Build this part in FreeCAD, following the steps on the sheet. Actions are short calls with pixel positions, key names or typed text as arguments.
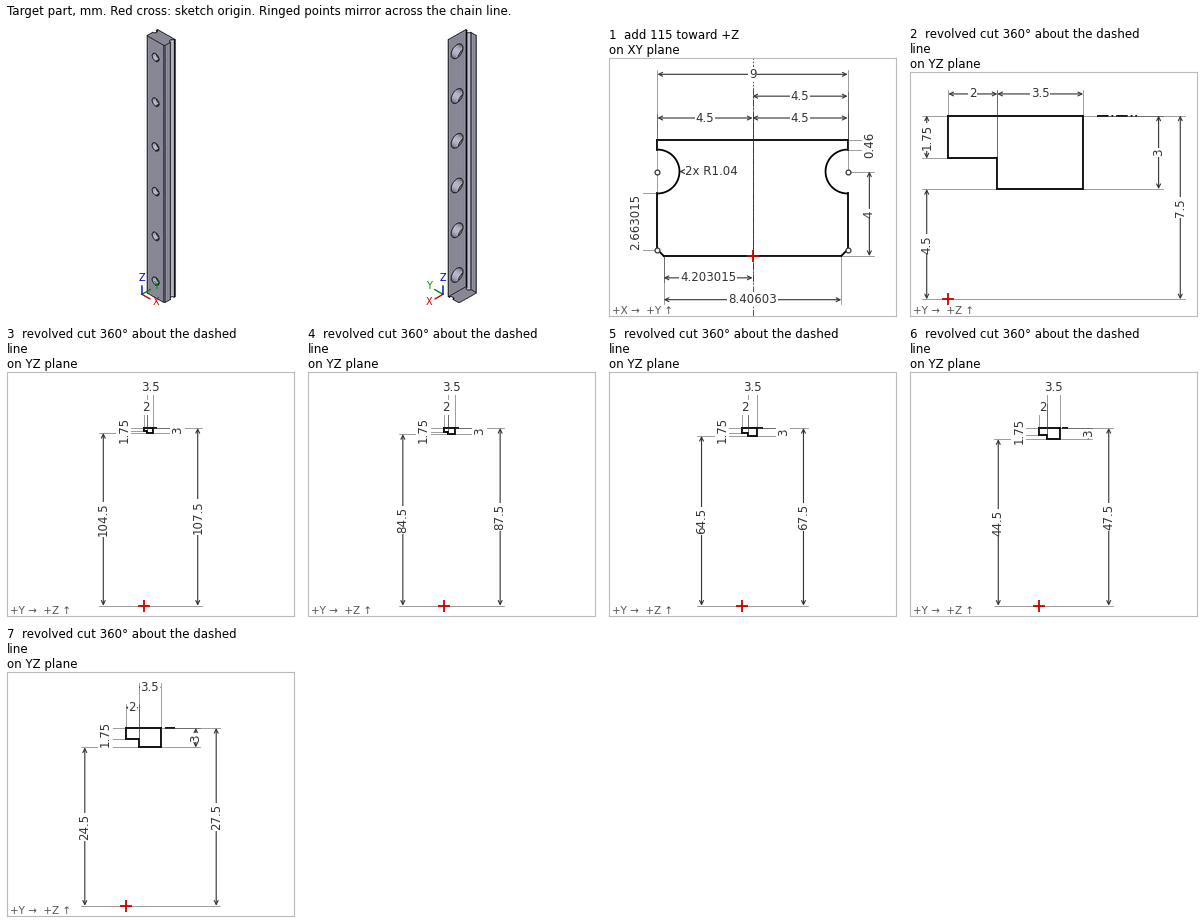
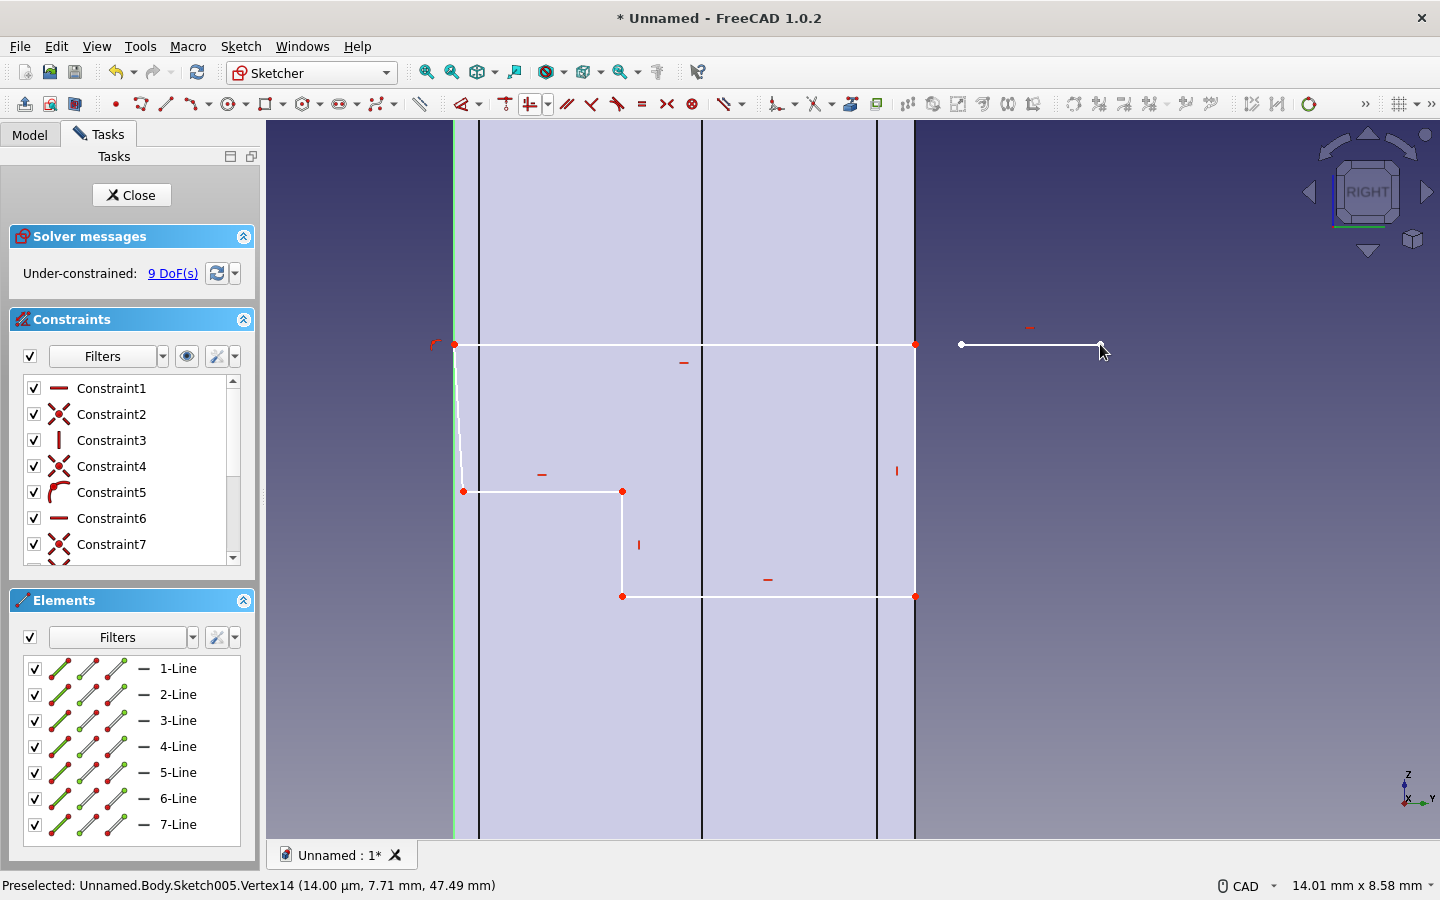
click(1003, 345)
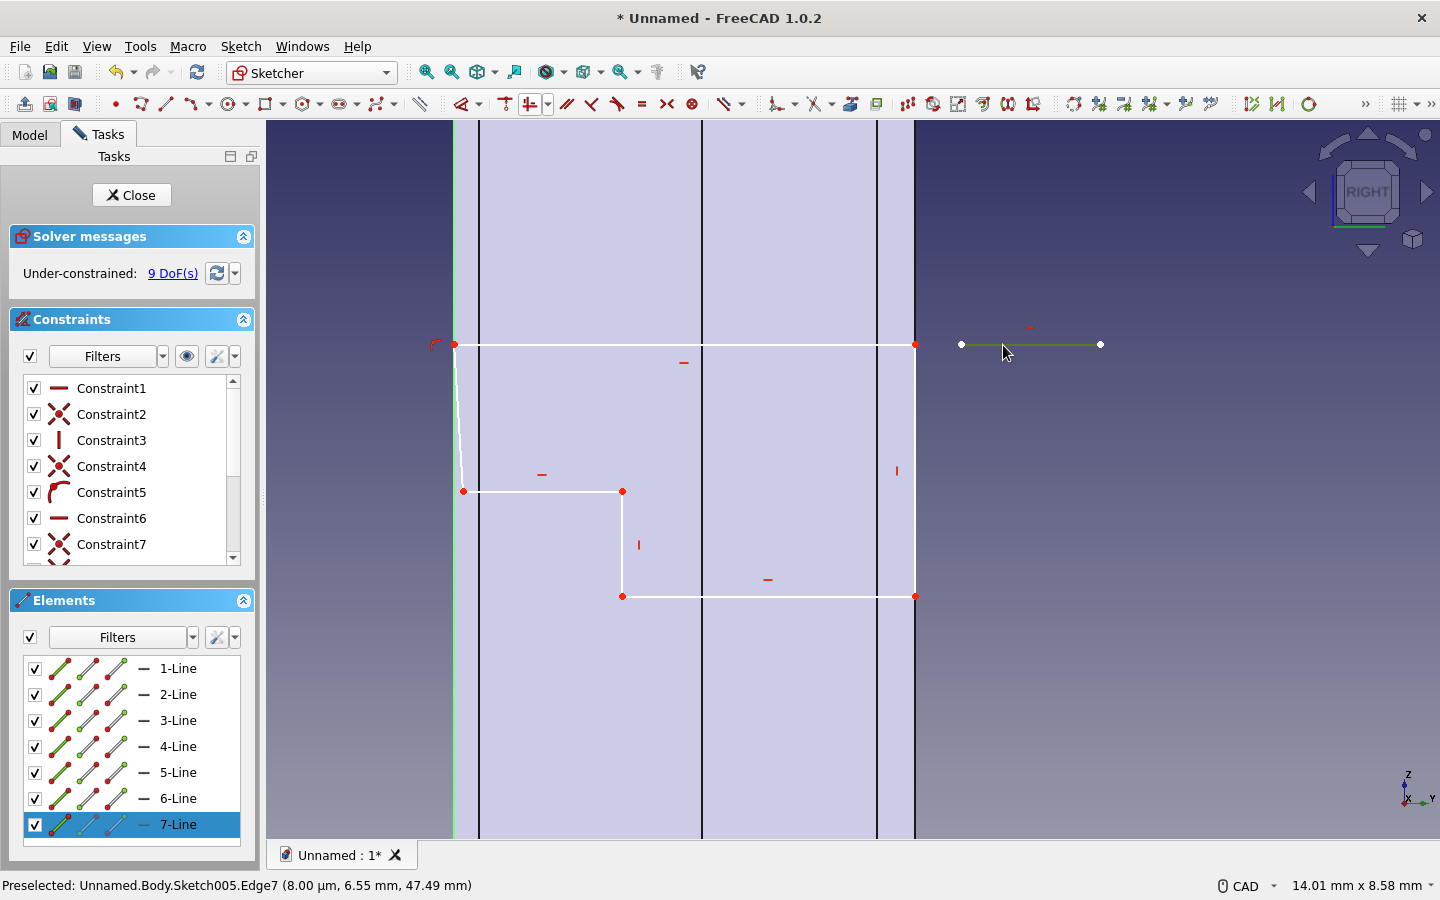
key(g)
key(n)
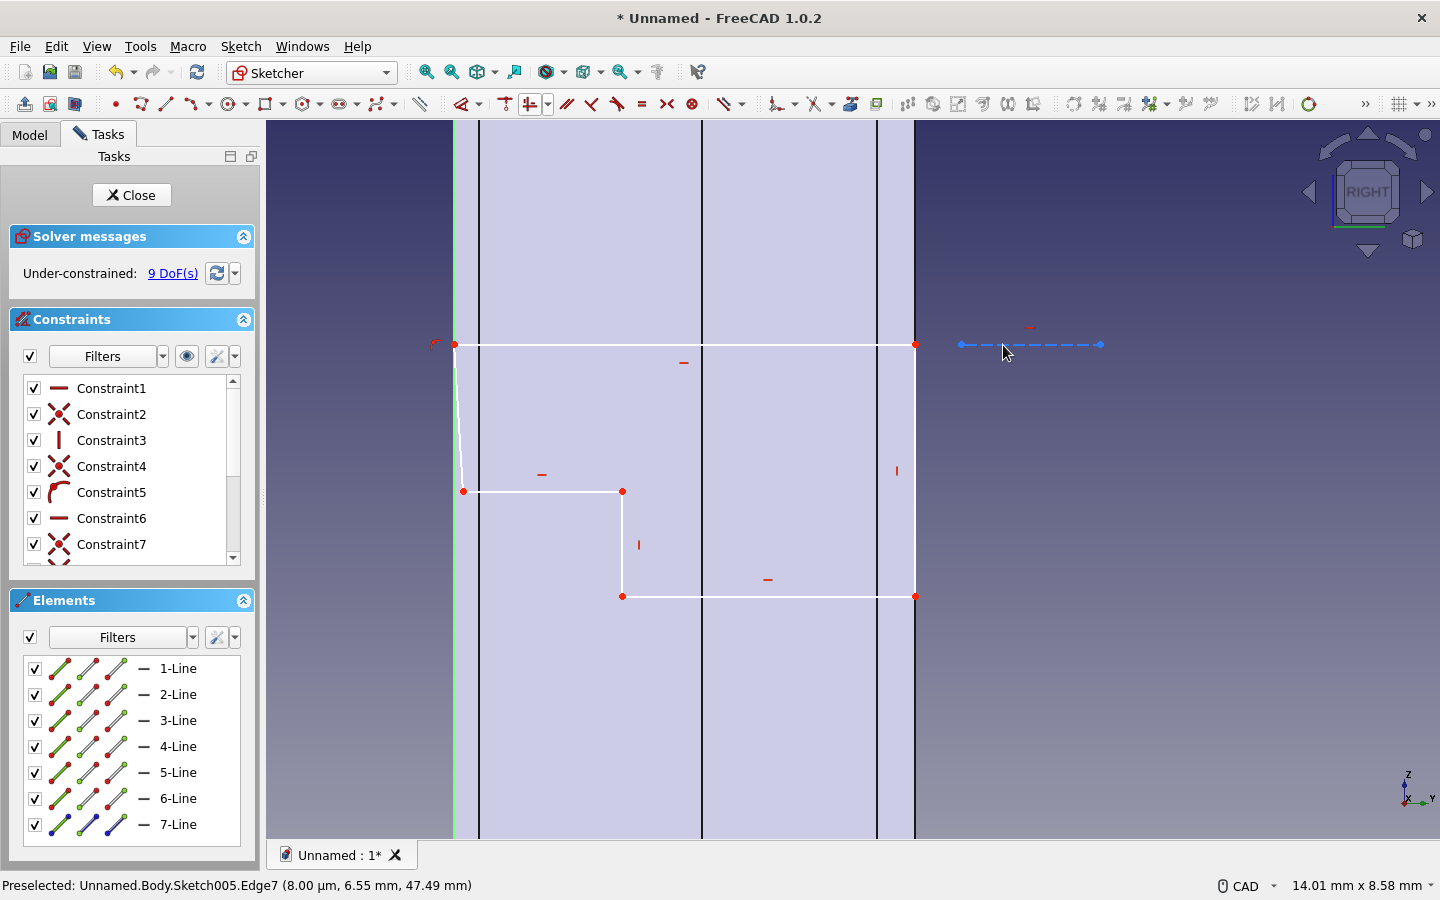
click(457, 389)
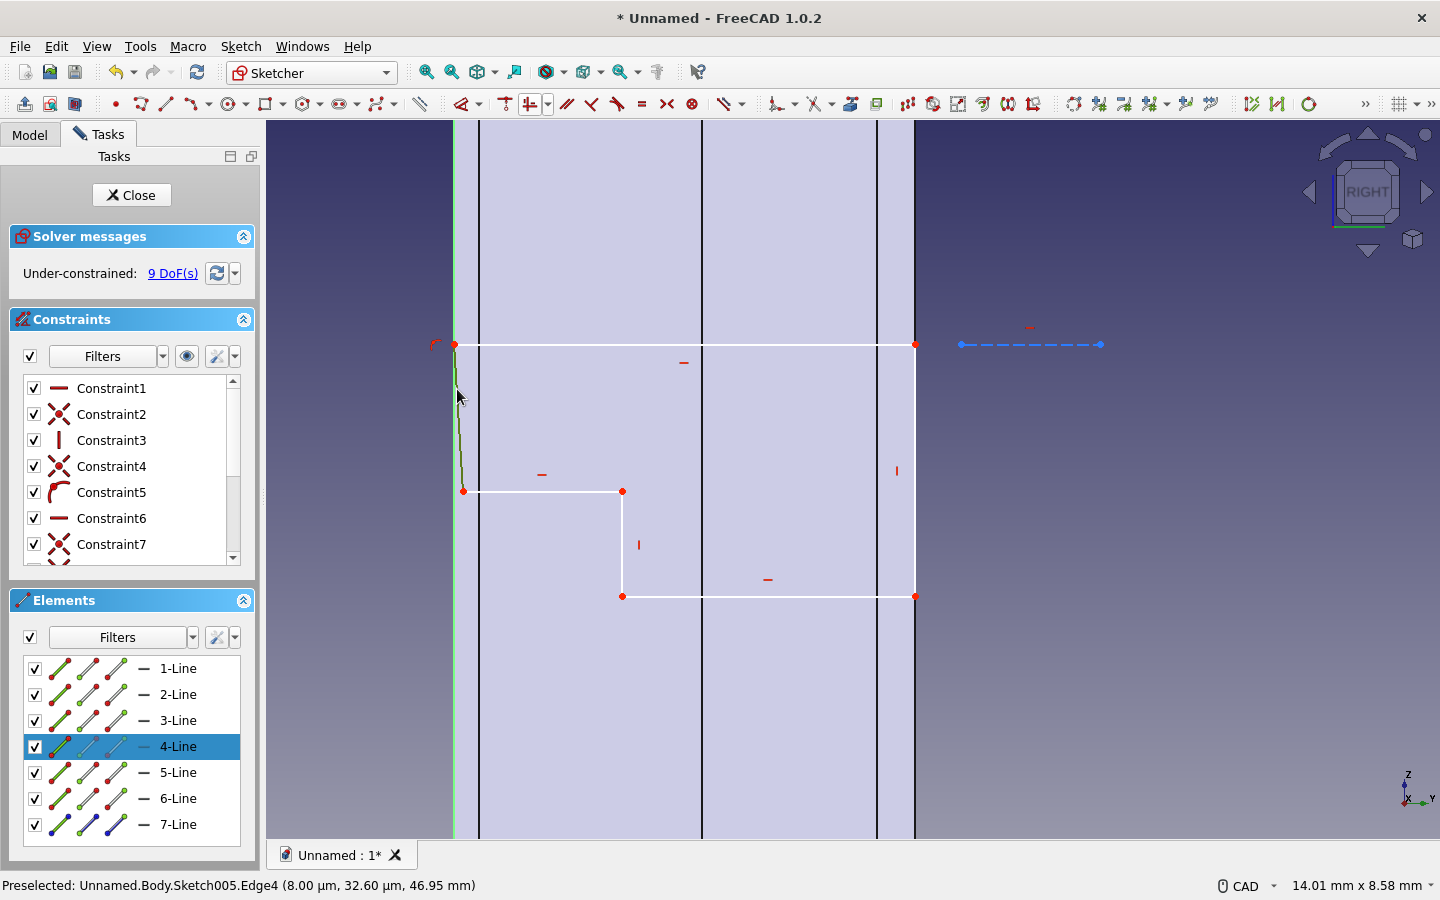
click(548, 104)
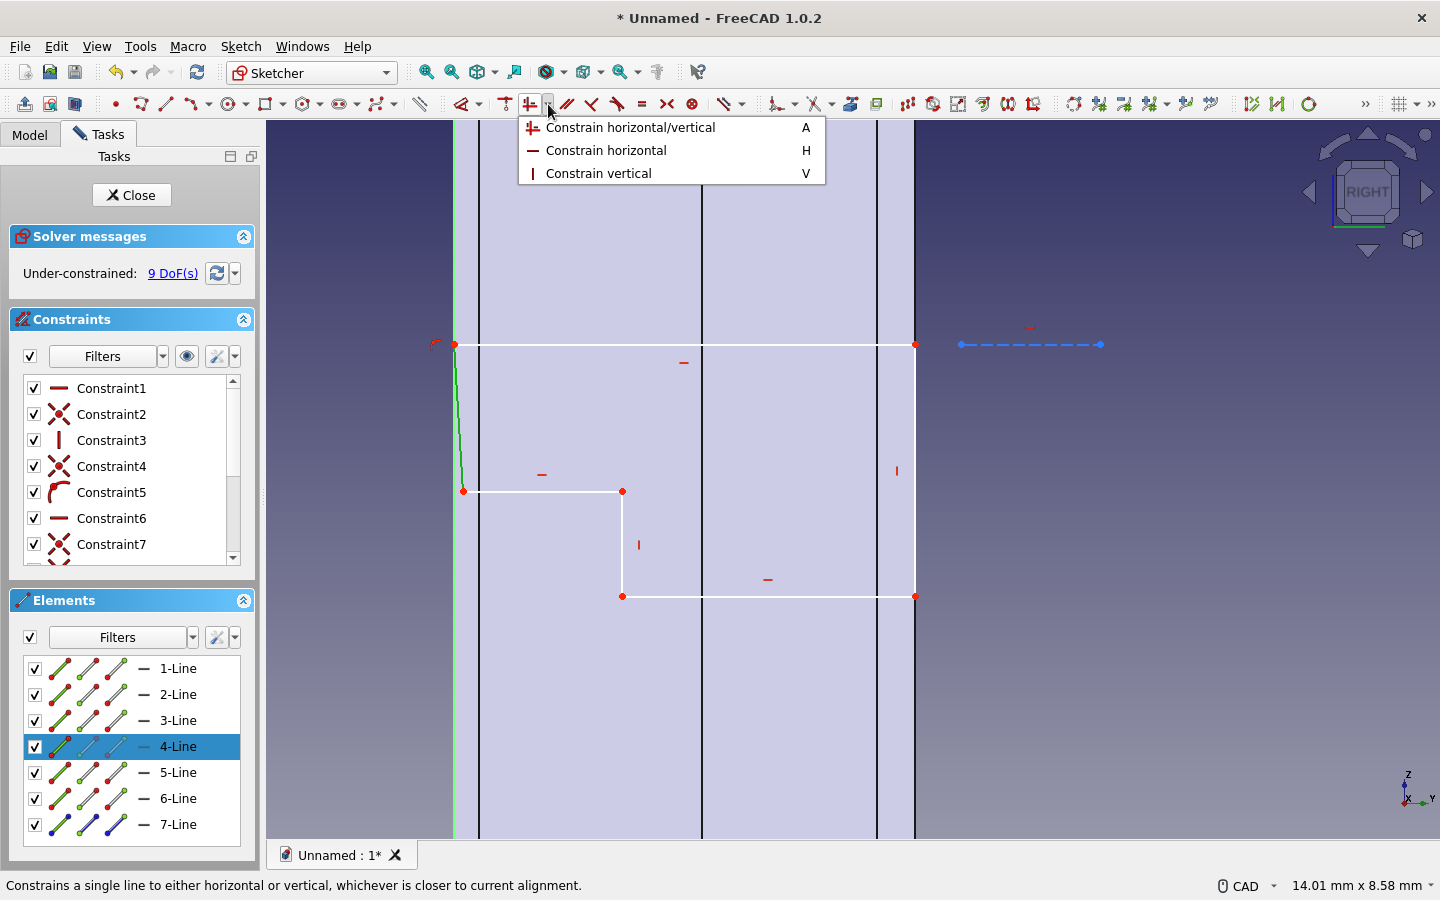
click(672, 174)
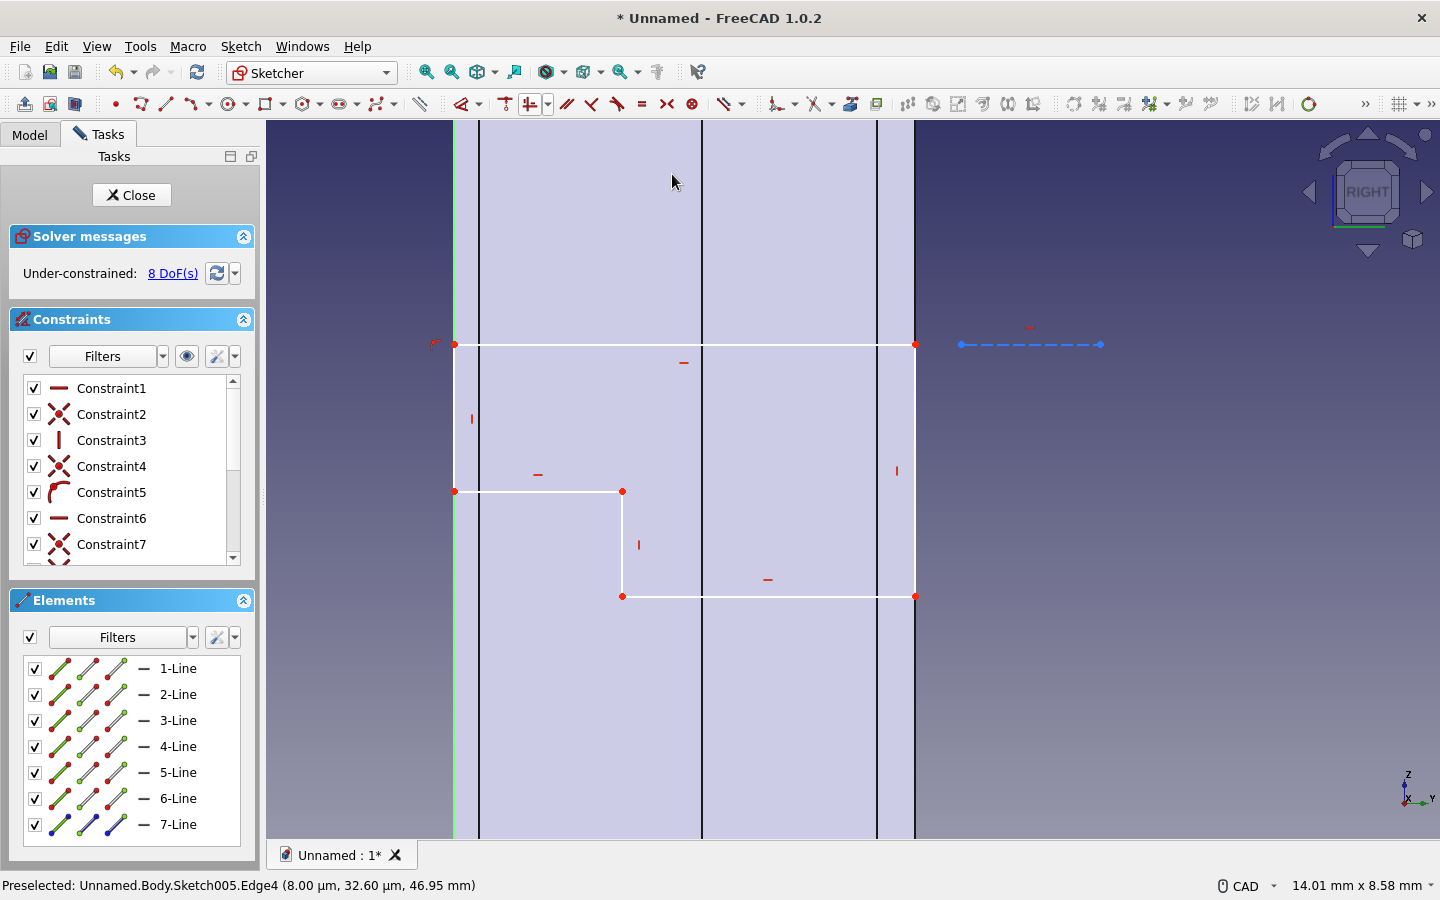
key(d)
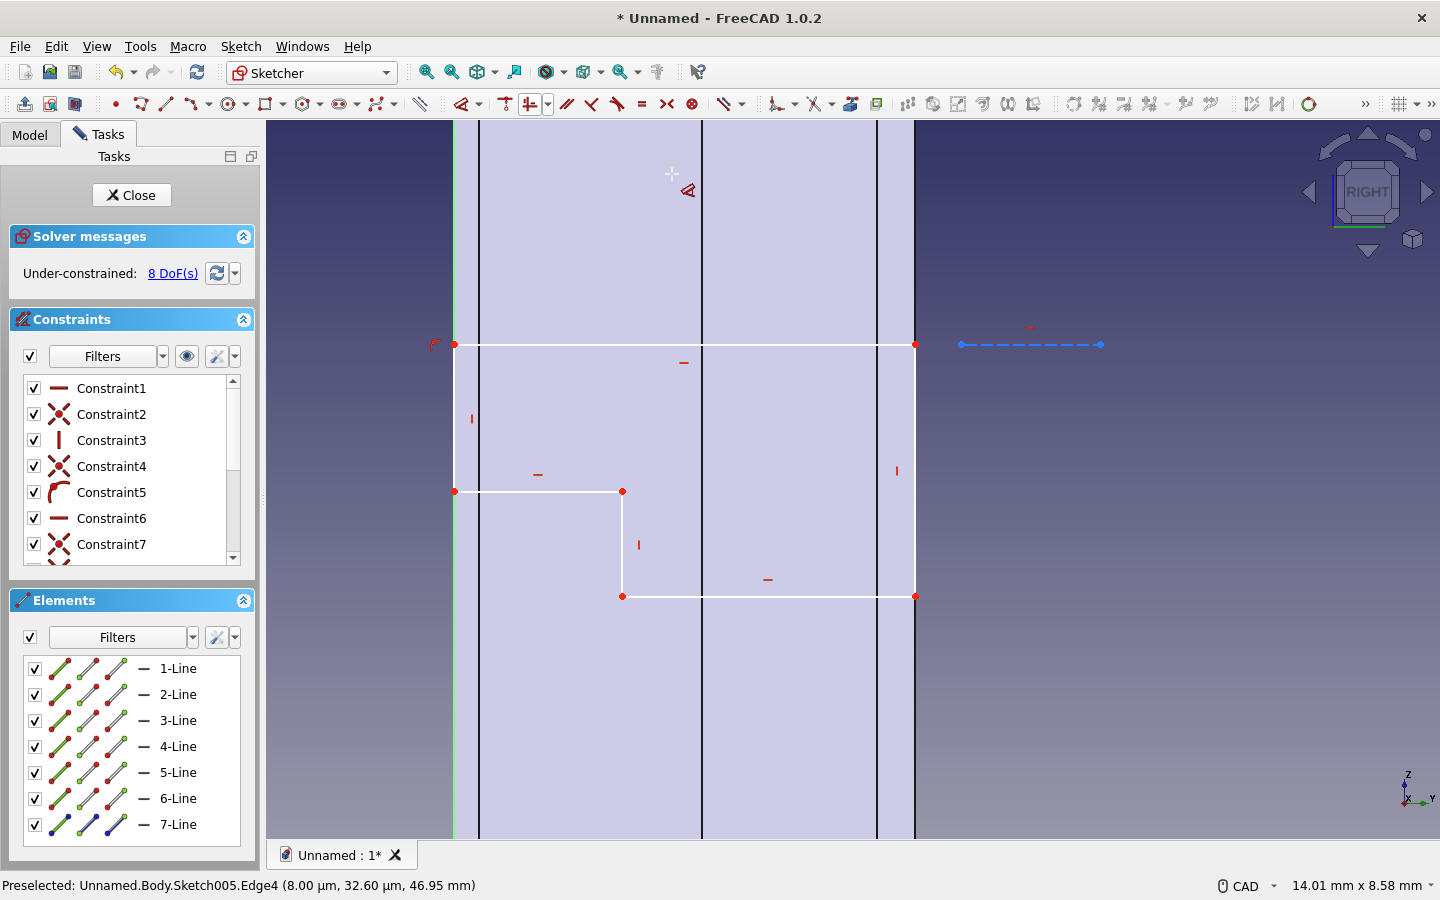
click(915, 521)
click(949, 471)